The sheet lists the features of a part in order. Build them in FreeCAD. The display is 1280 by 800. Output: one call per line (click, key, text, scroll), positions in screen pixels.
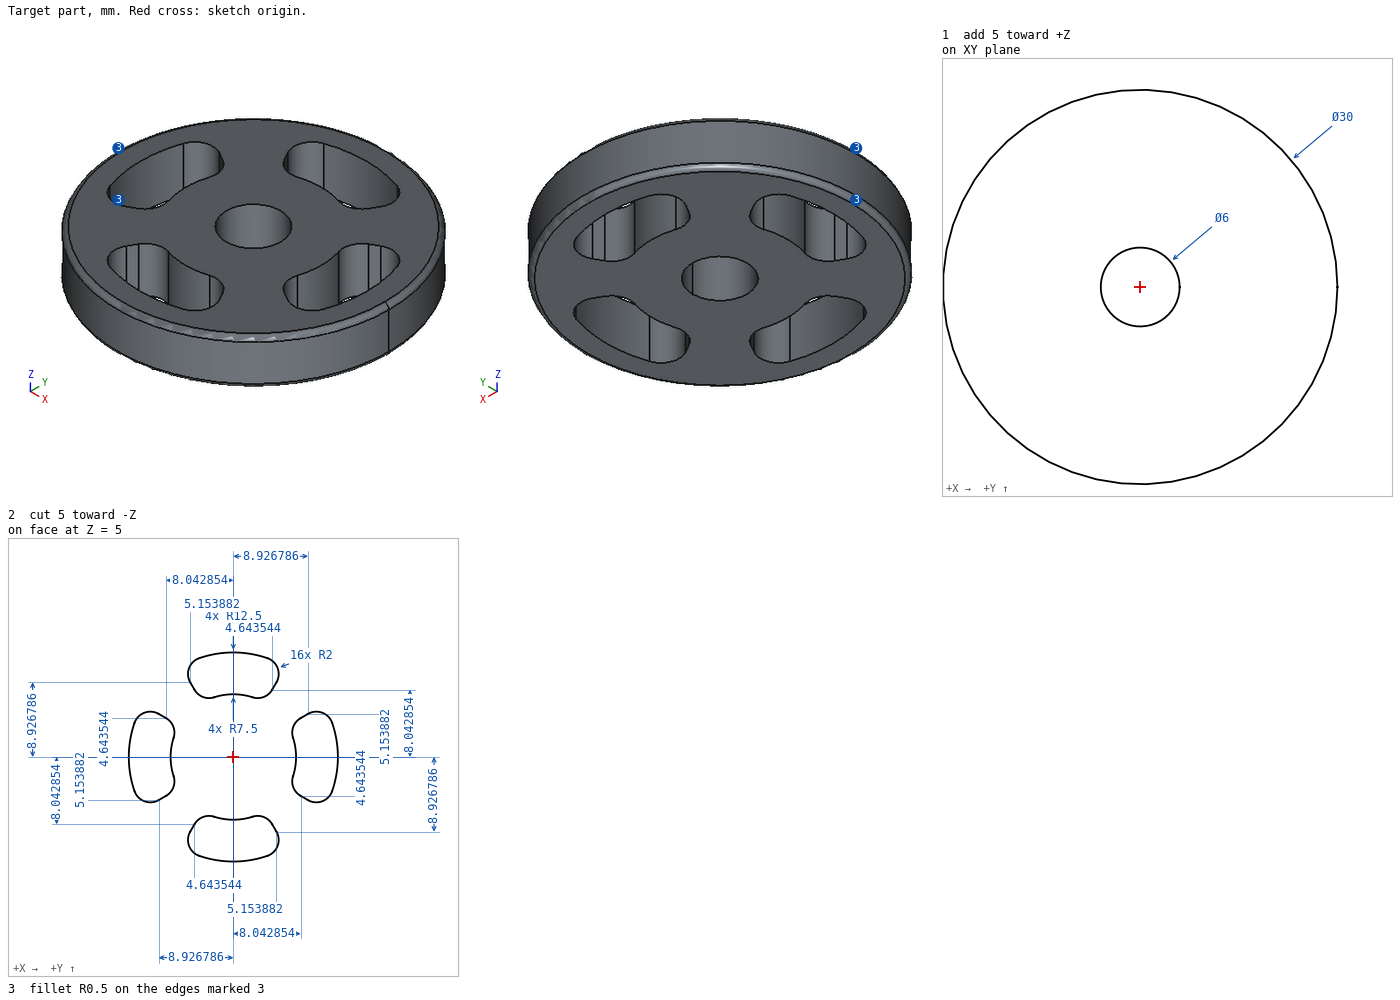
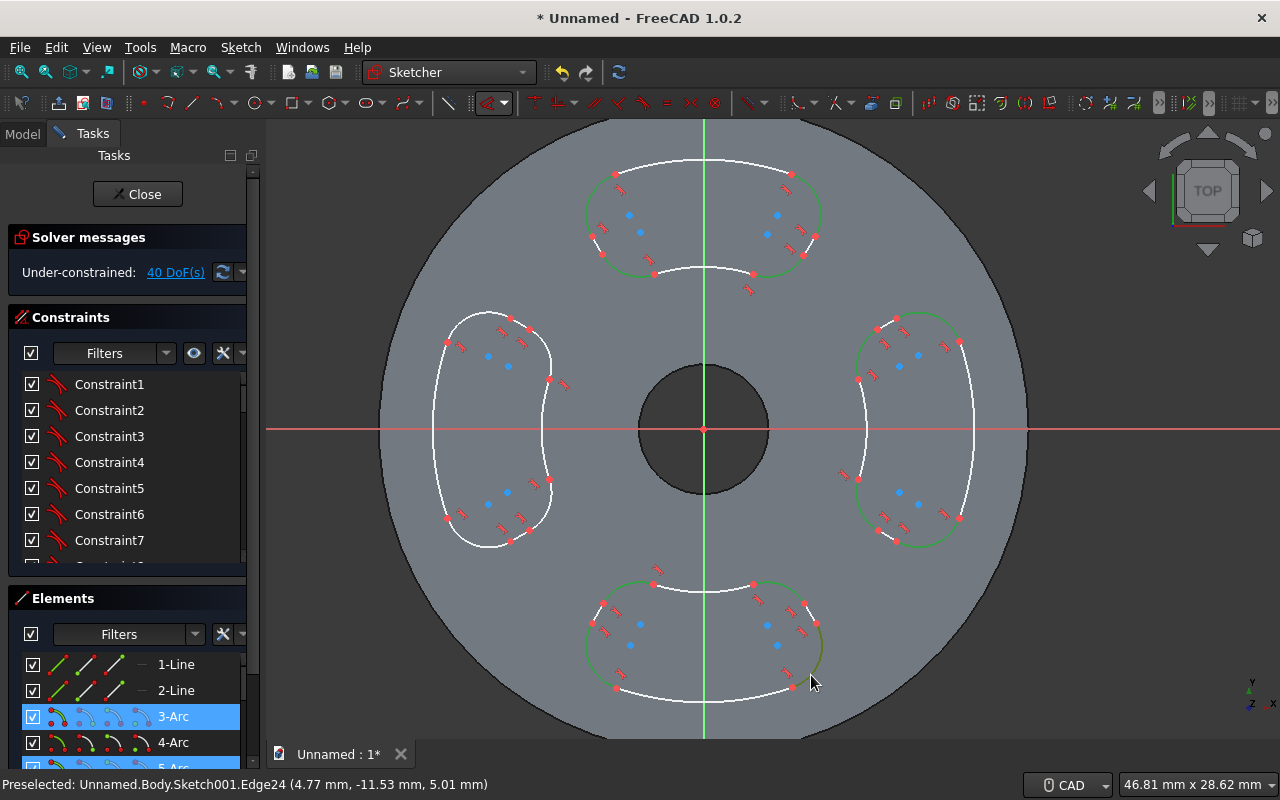
click(543, 519)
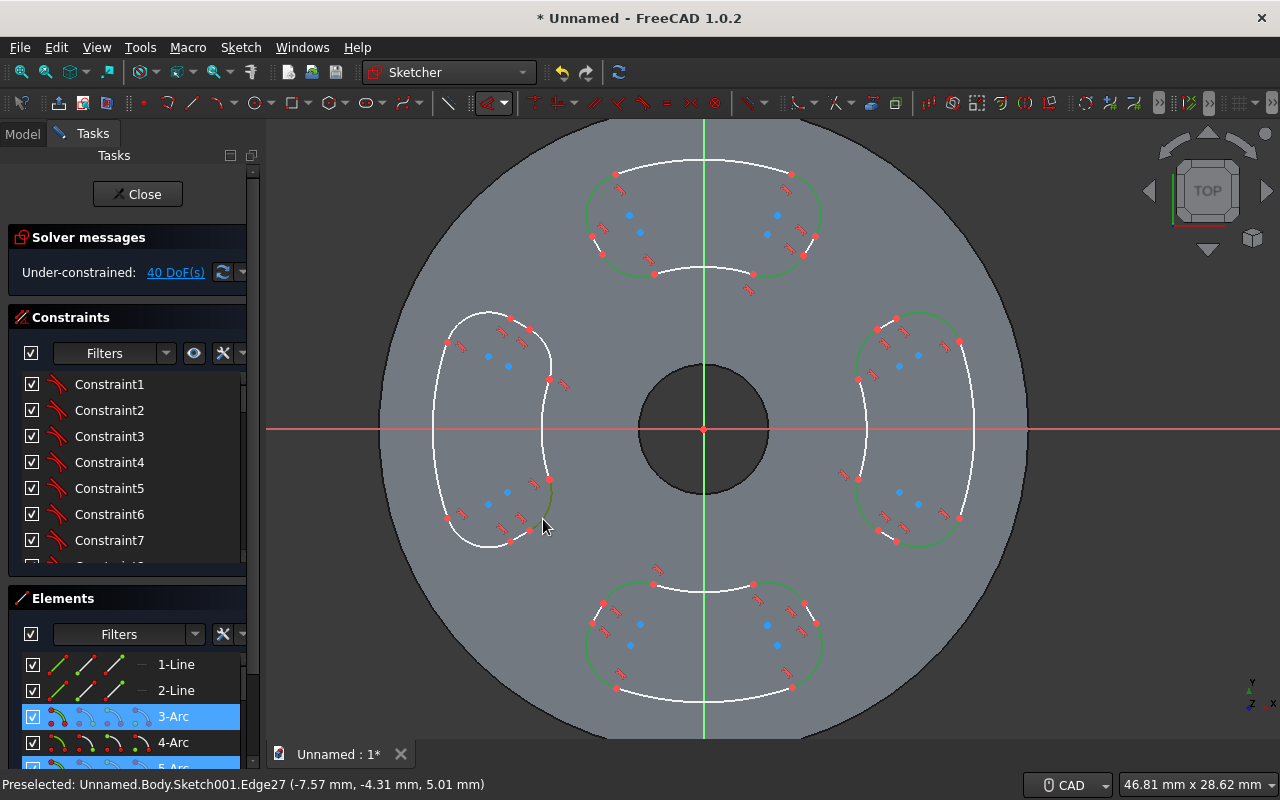
click(551, 363)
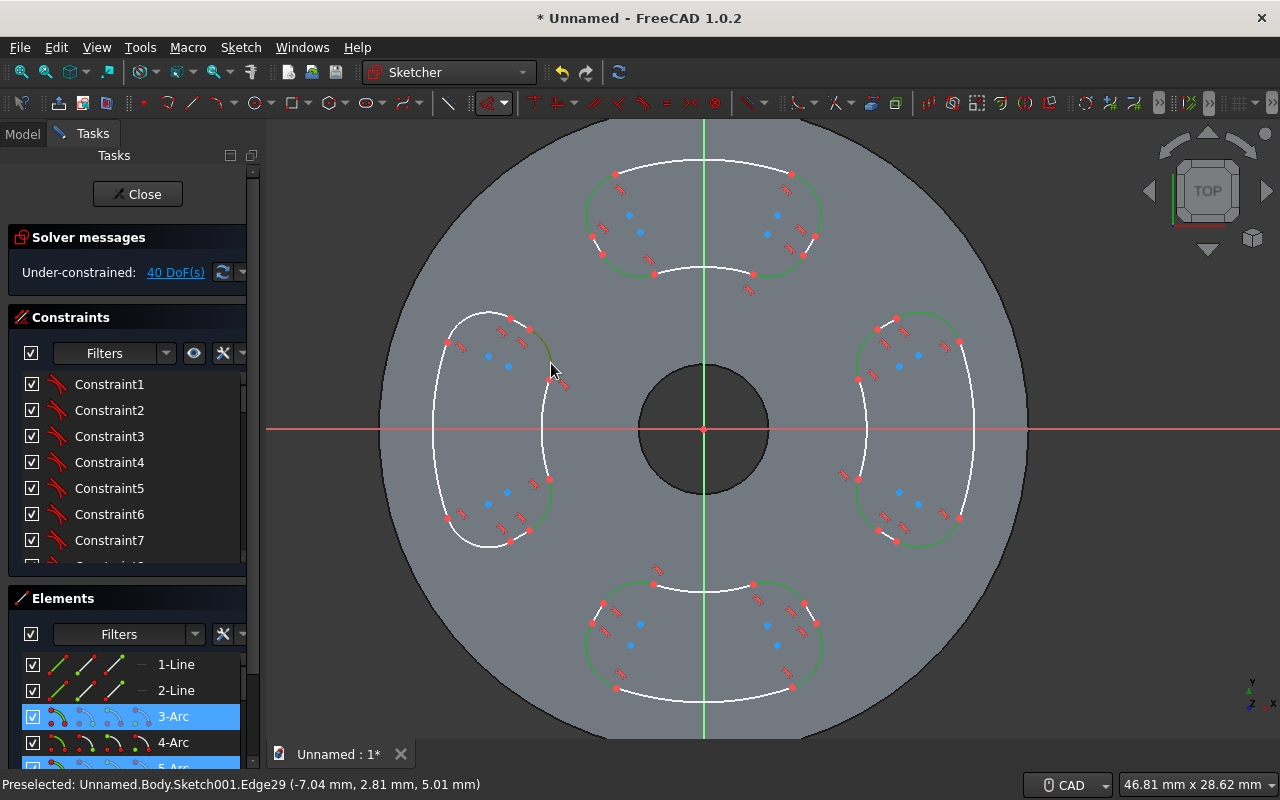
click(488, 312)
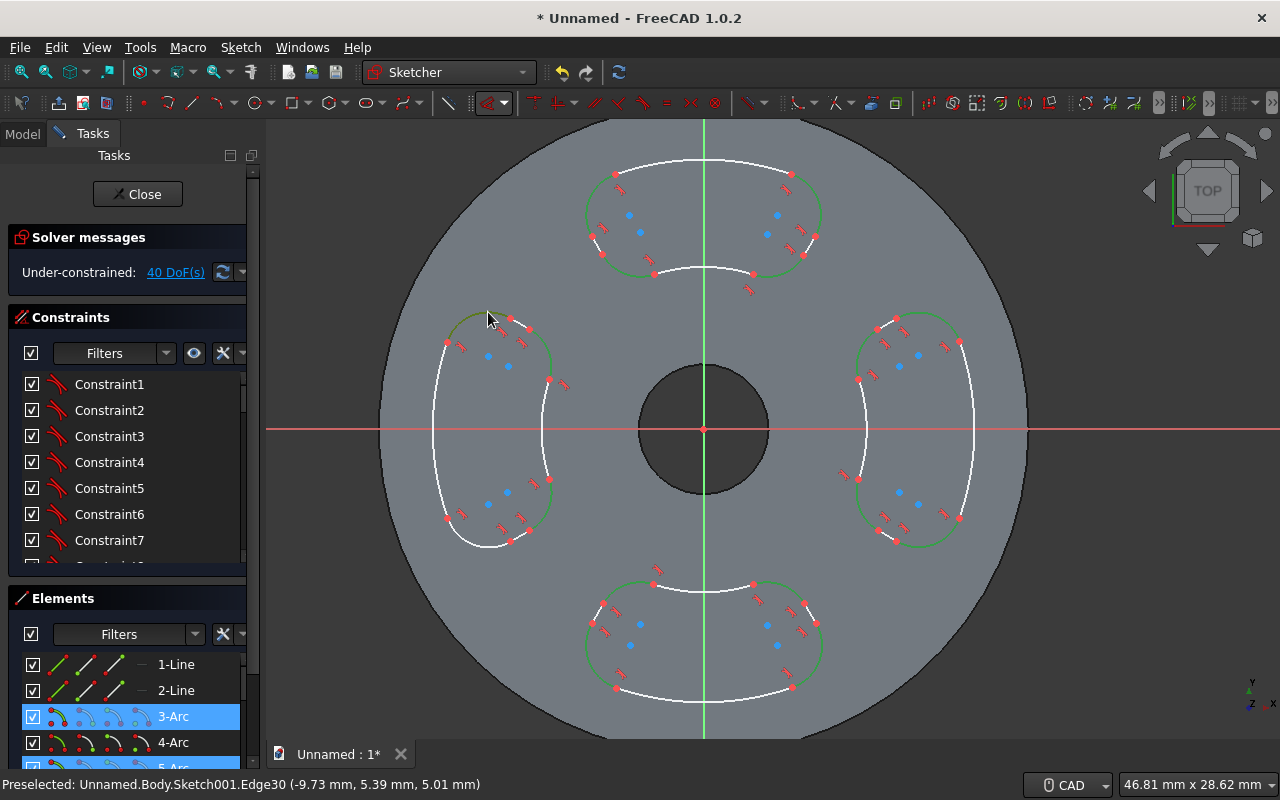
click(461, 537)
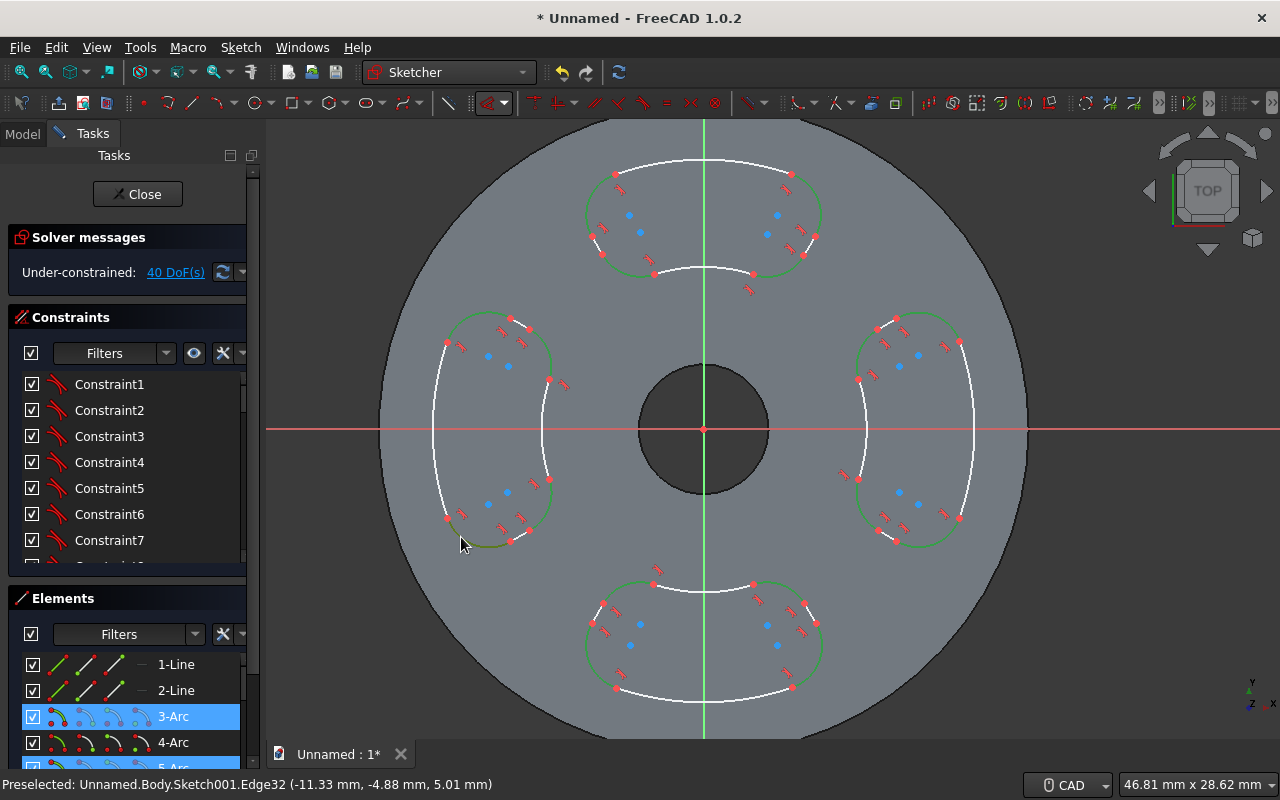
click(668, 104)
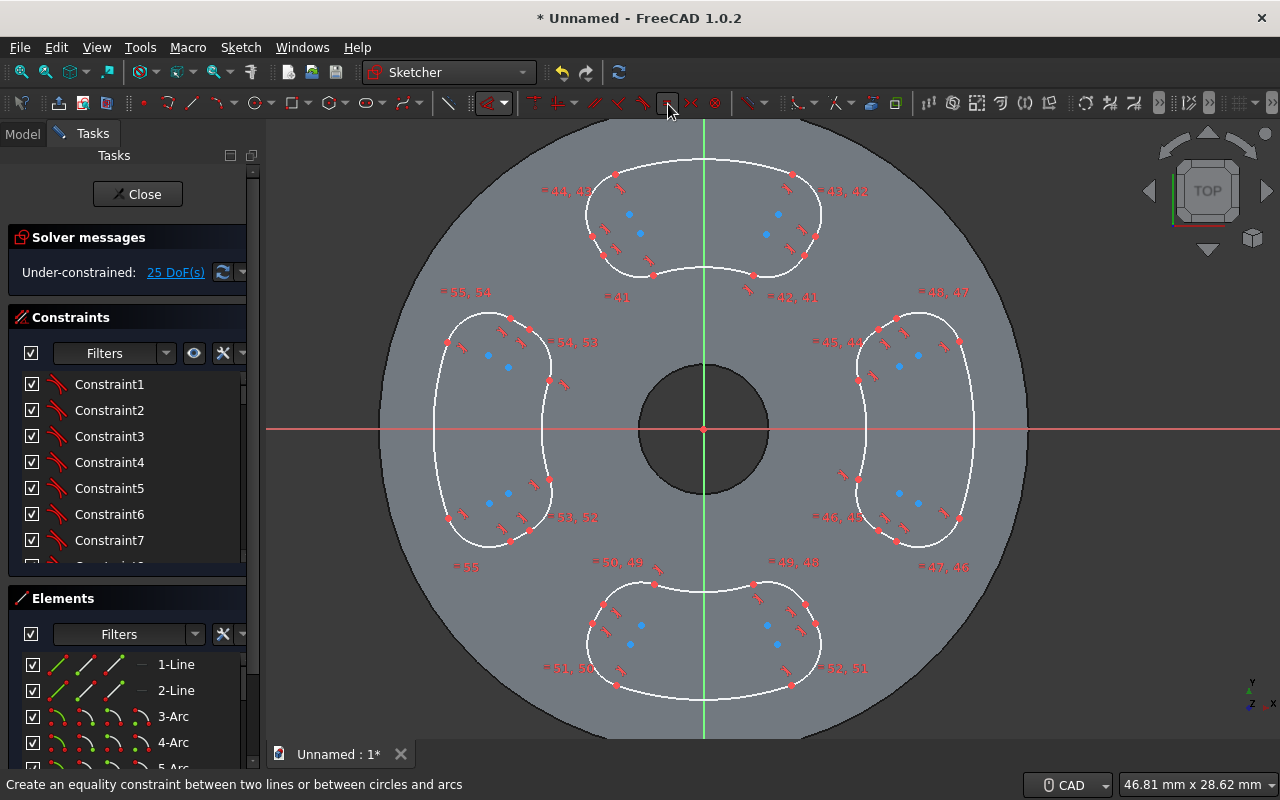
click(724, 269)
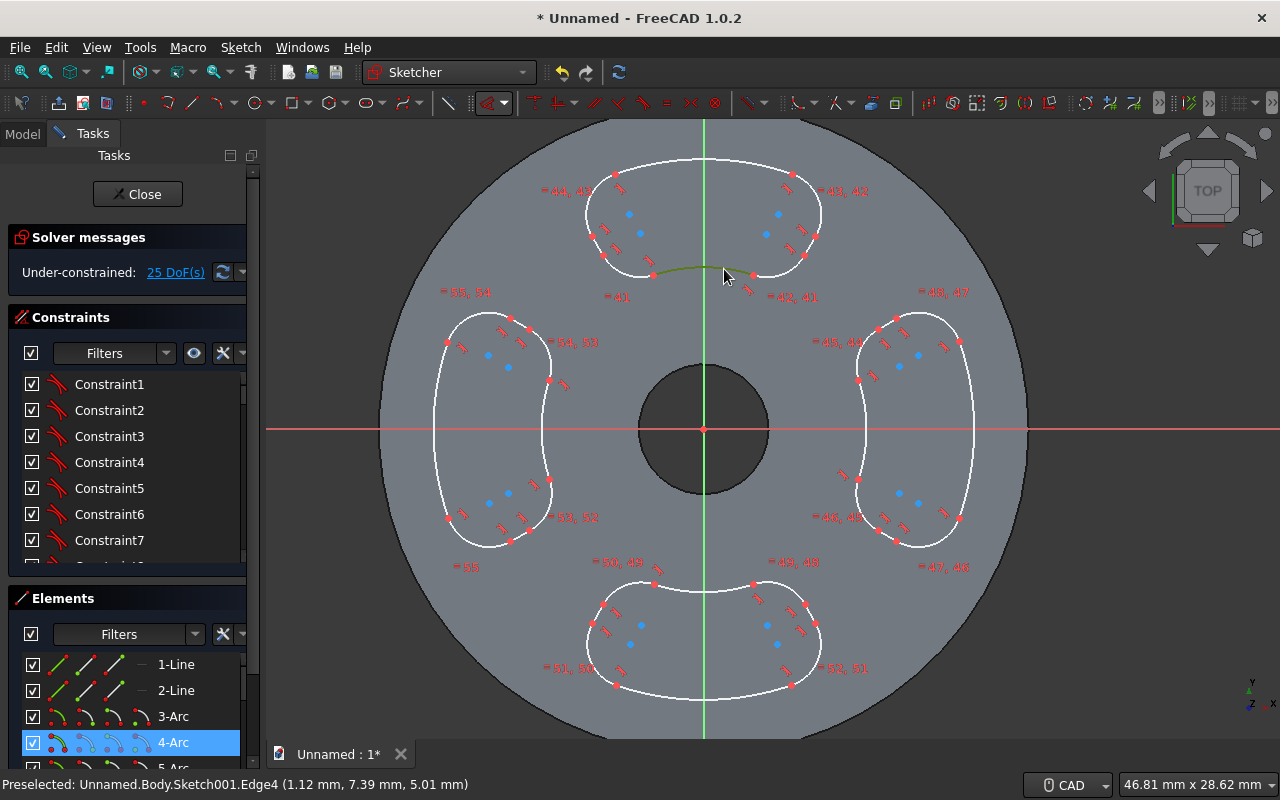
click(865, 450)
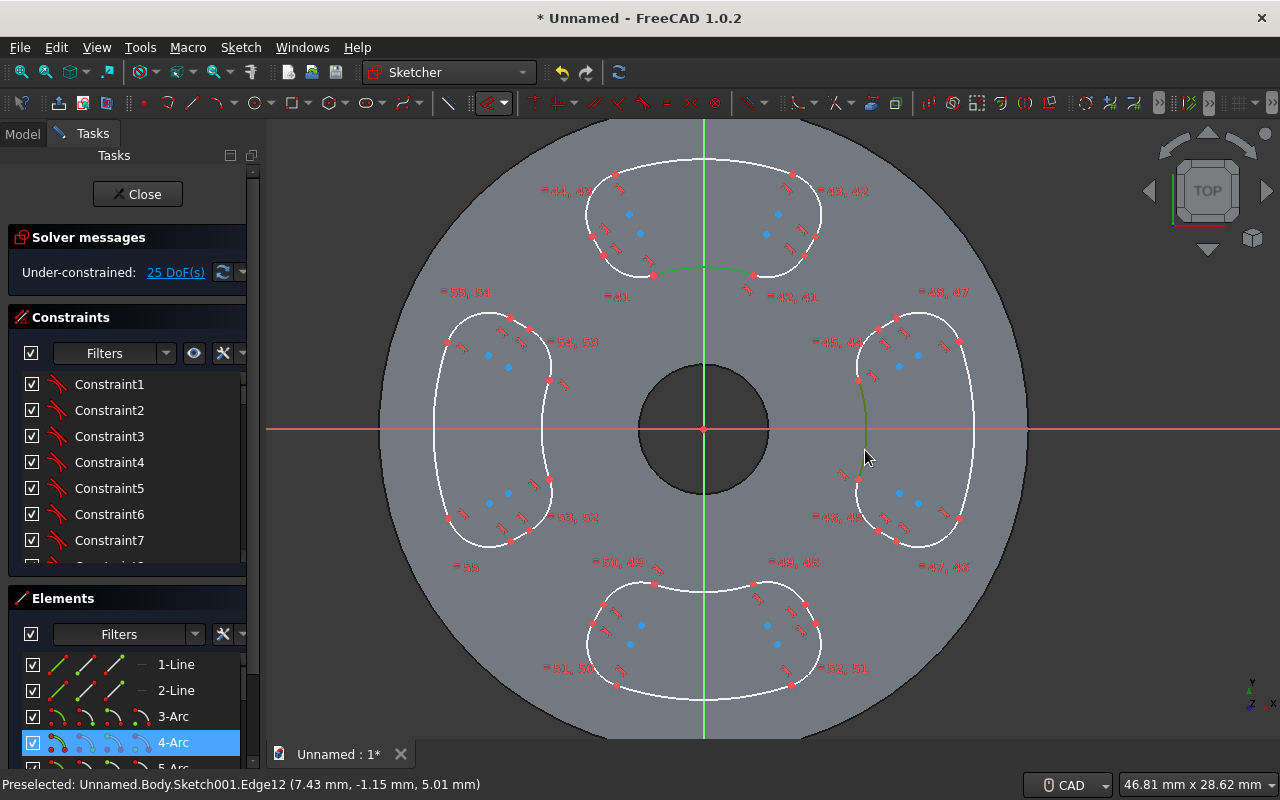
click(684, 591)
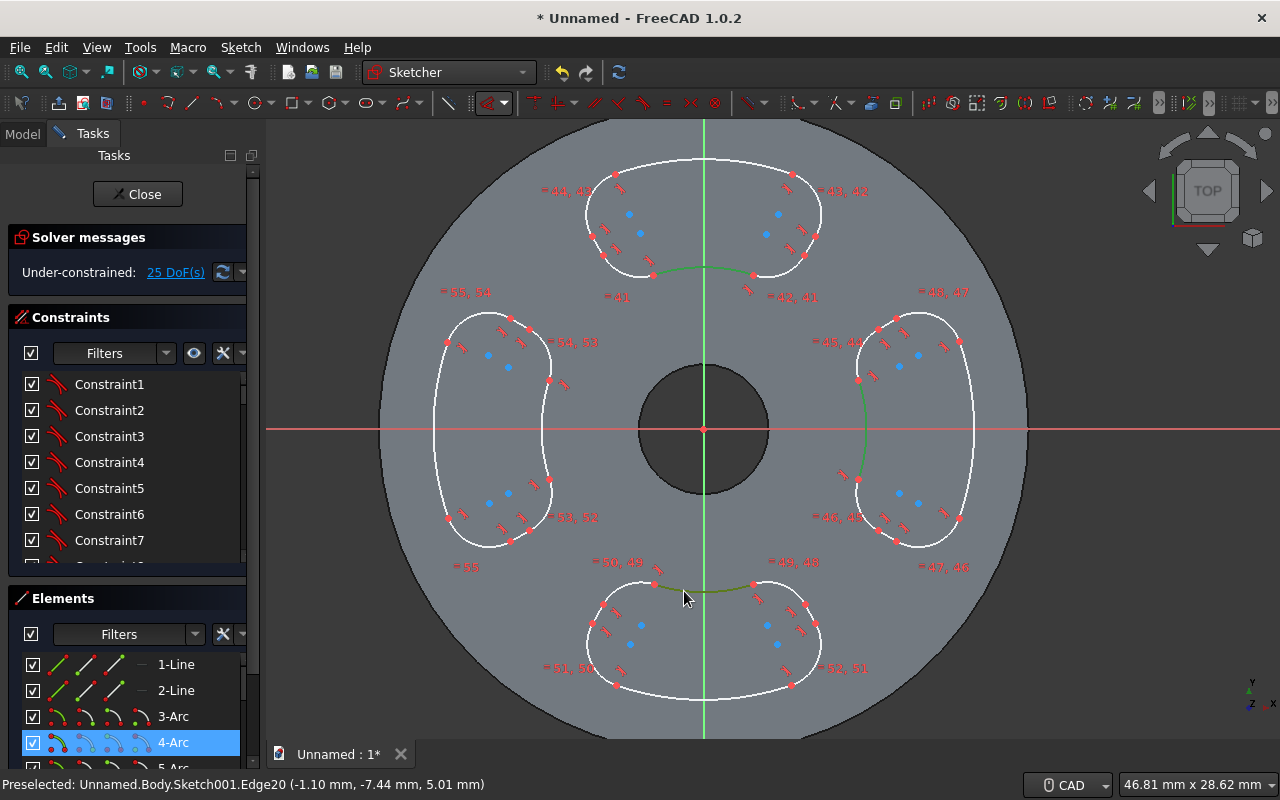
click(543, 410)